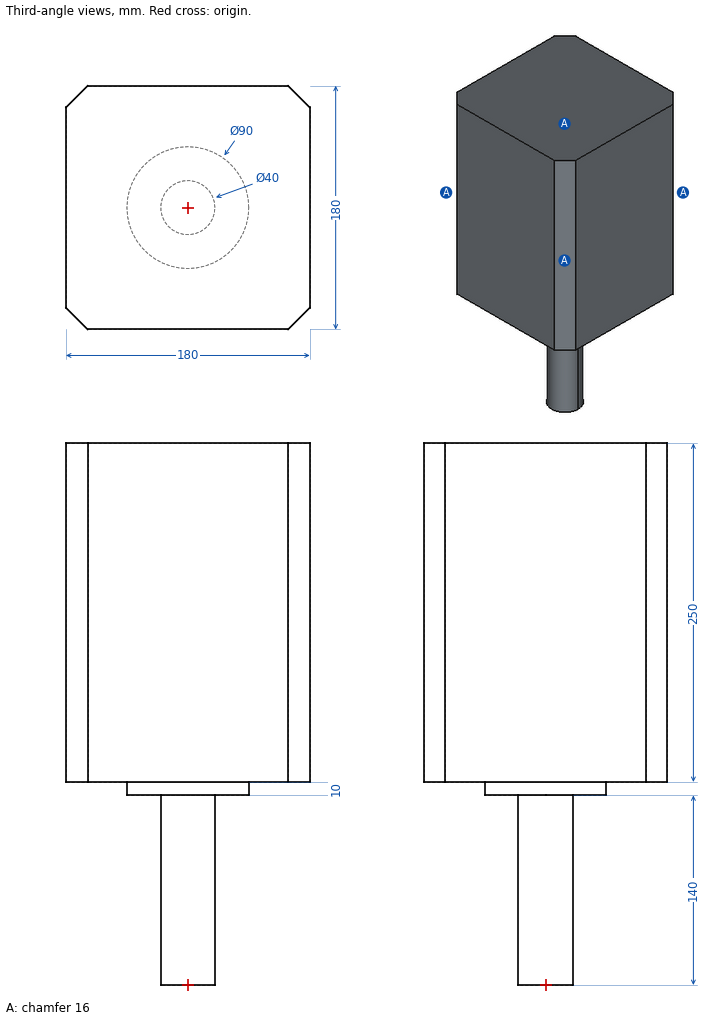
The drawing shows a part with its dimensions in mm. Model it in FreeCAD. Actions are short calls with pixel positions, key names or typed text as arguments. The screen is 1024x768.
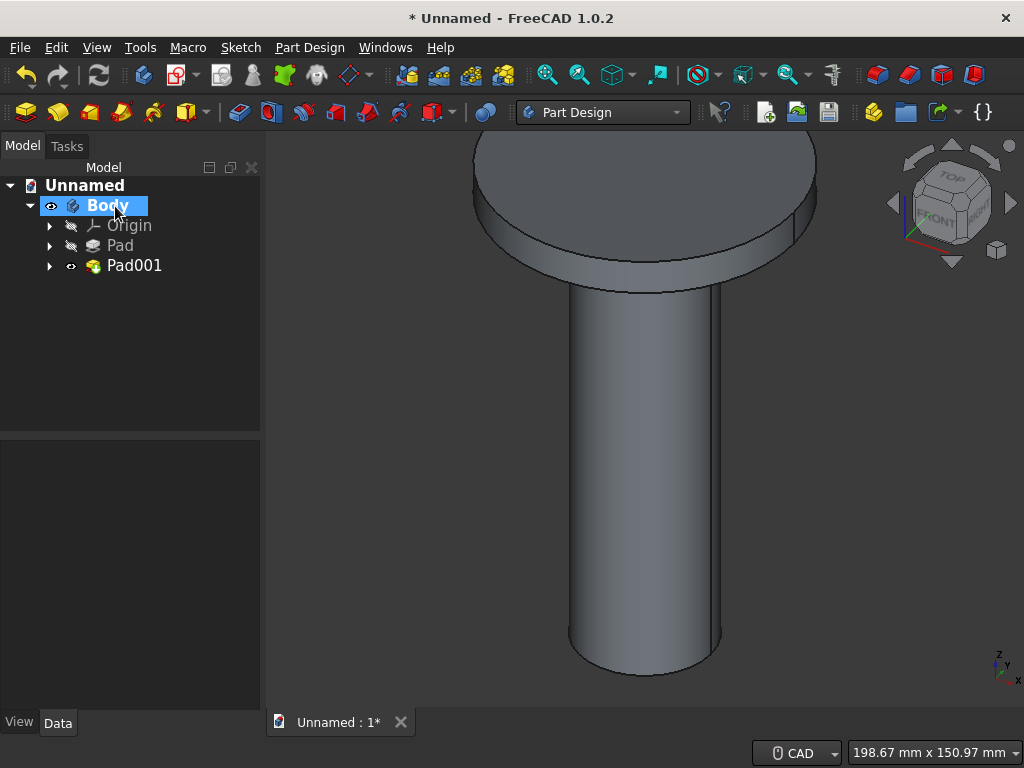
click(548, 76)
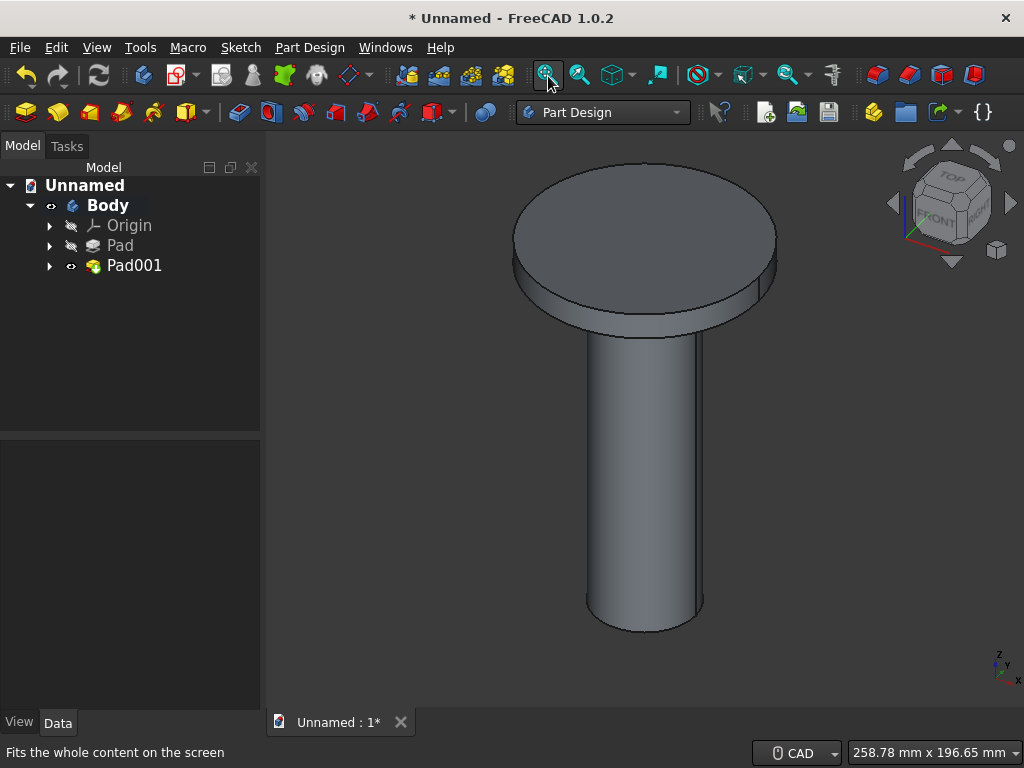
click(645, 238)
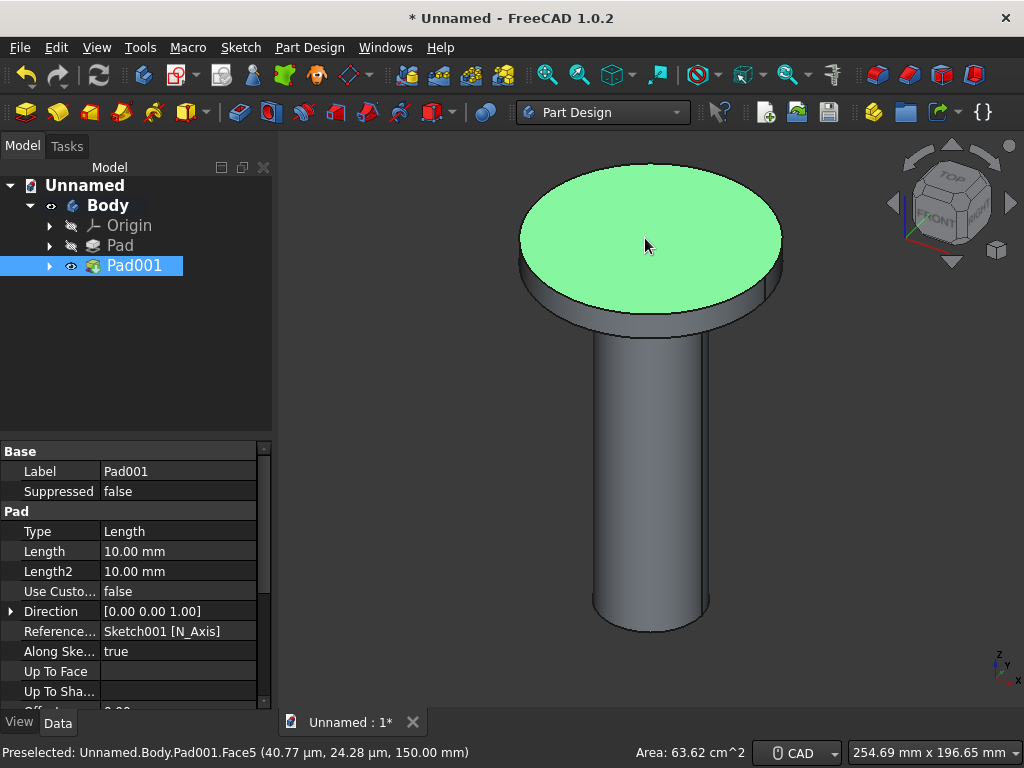
click(176, 76)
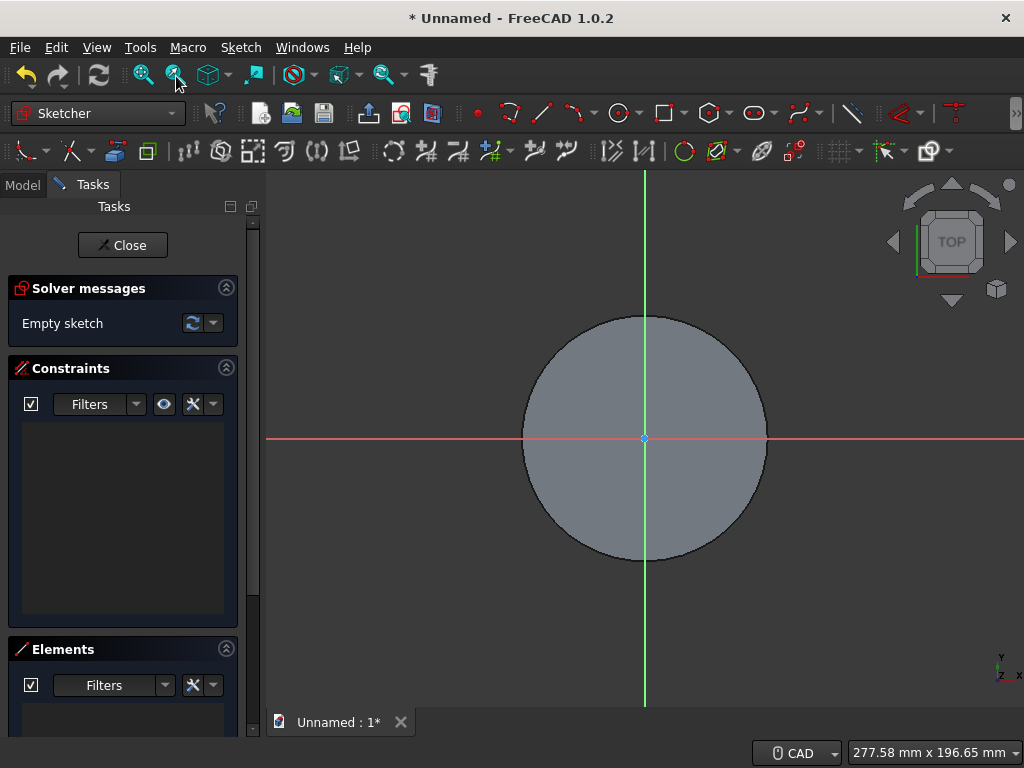
scroll(438, 438, down, 2)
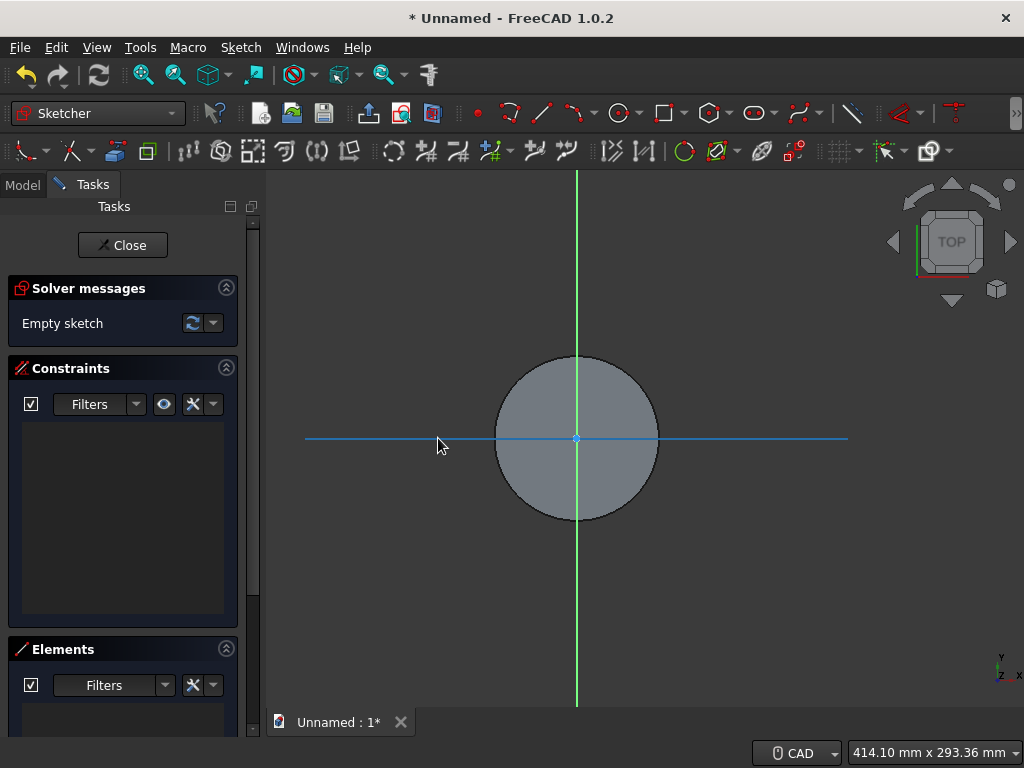
key(g)
key(v)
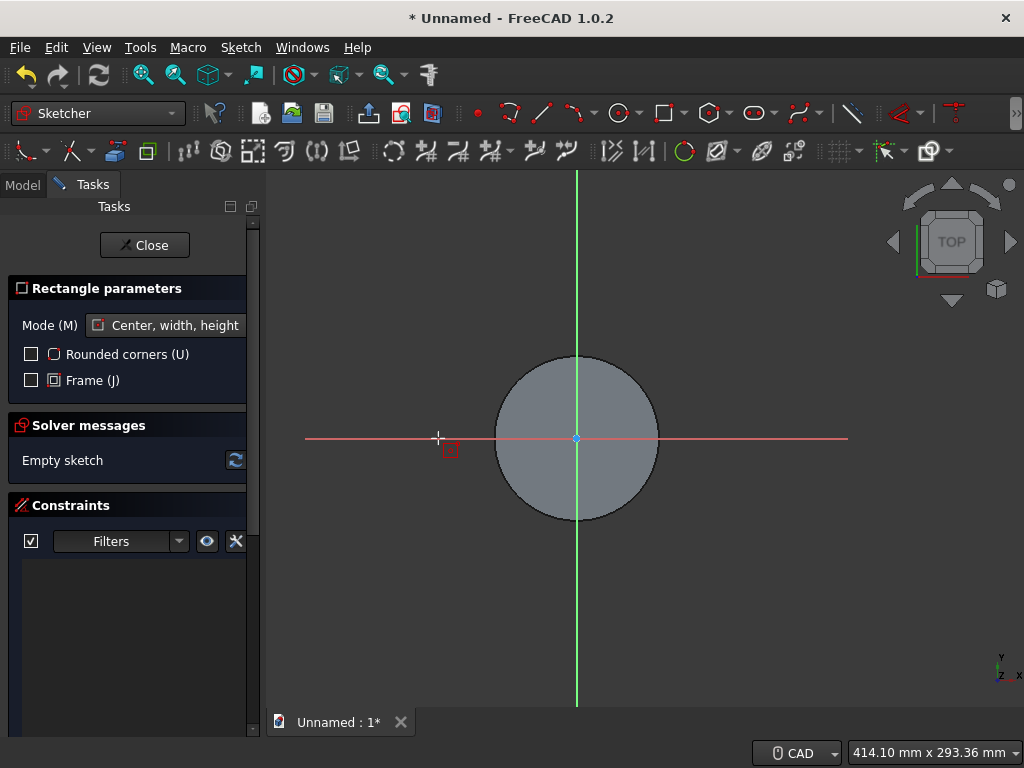
click(577, 438)
click(741, 274)
key(Escape)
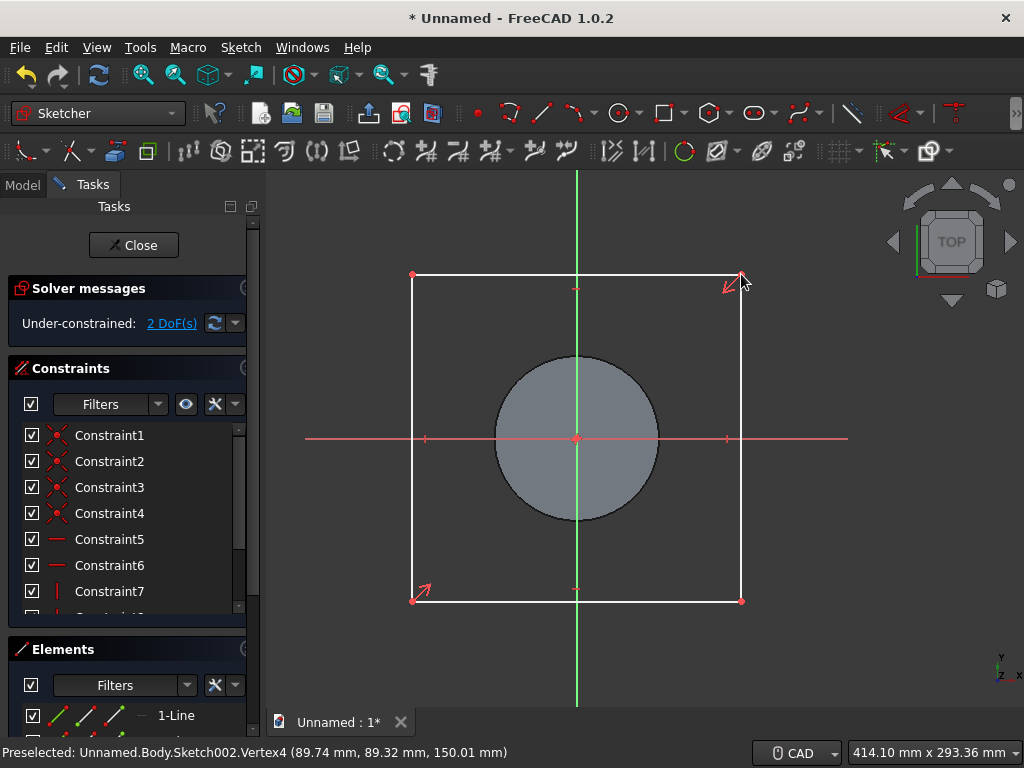
click(900, 114)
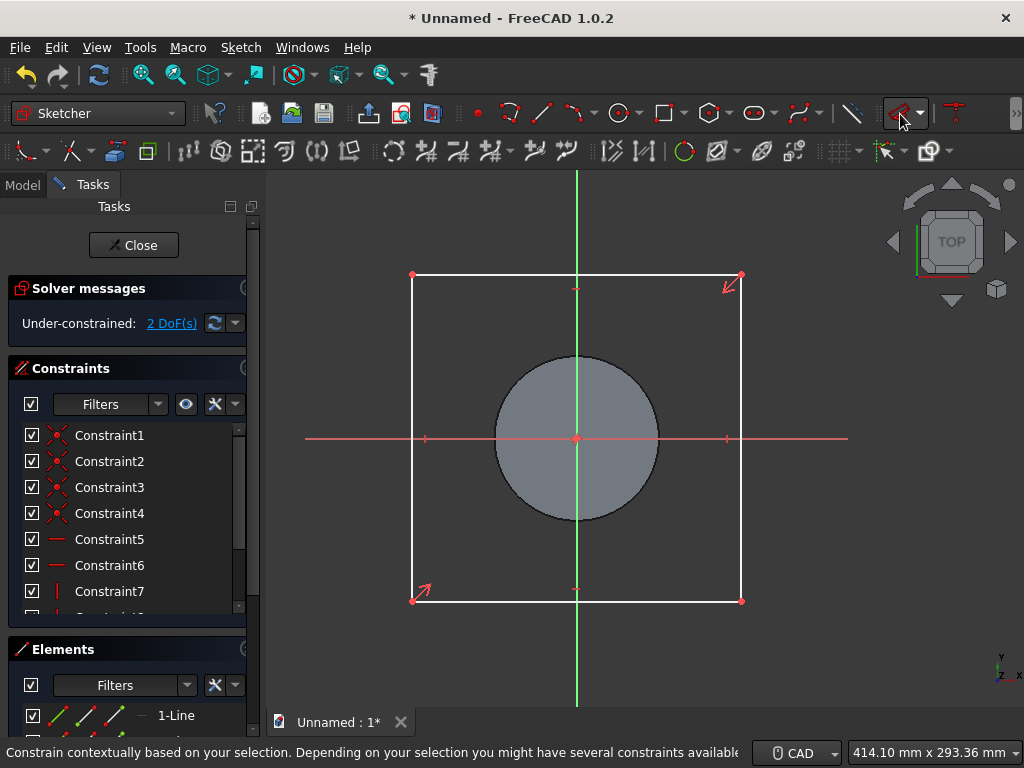
click(511, 602)
click(501, 636)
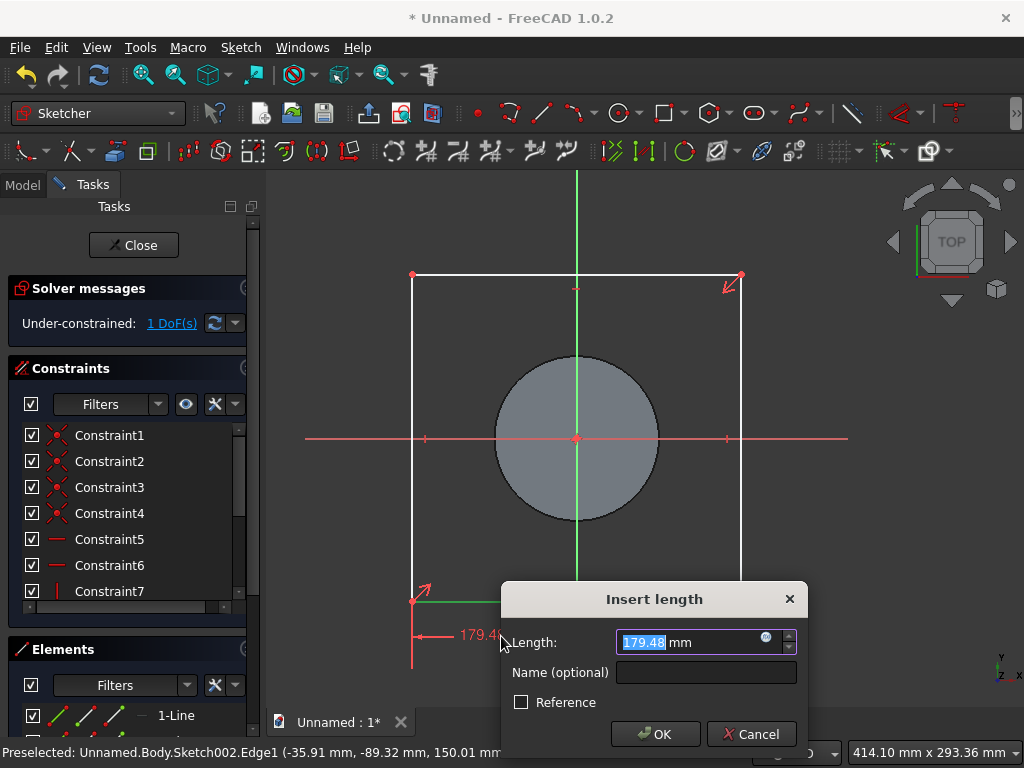
text(180)
key(Return)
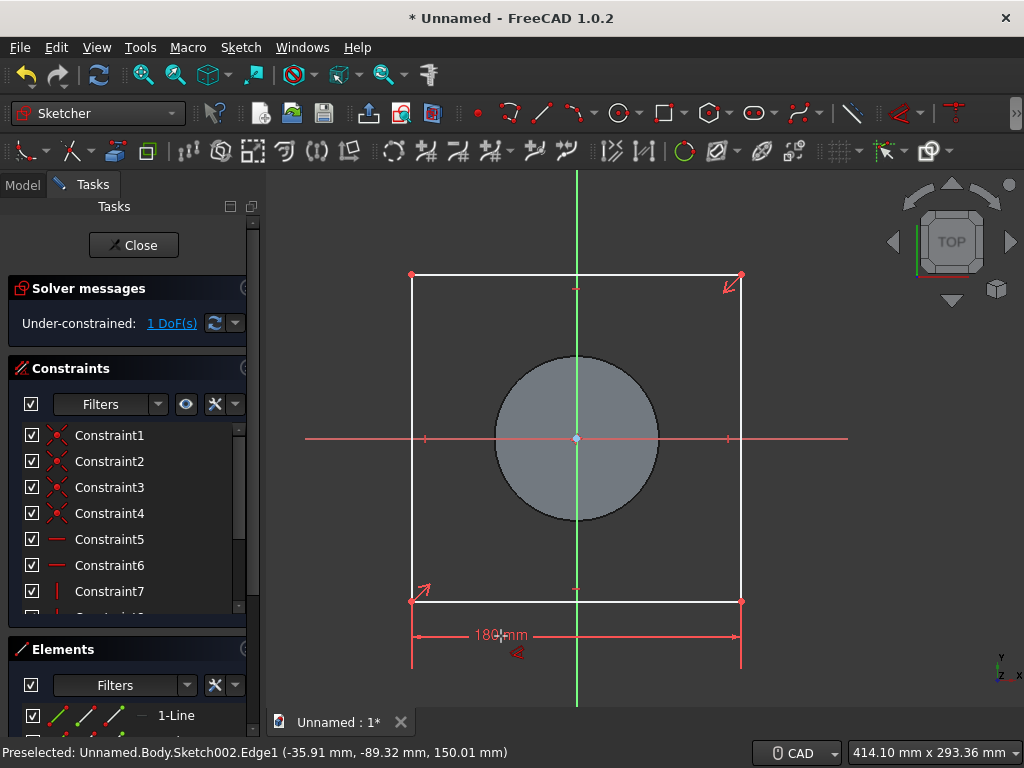
click(741, 504)
click(775, 363)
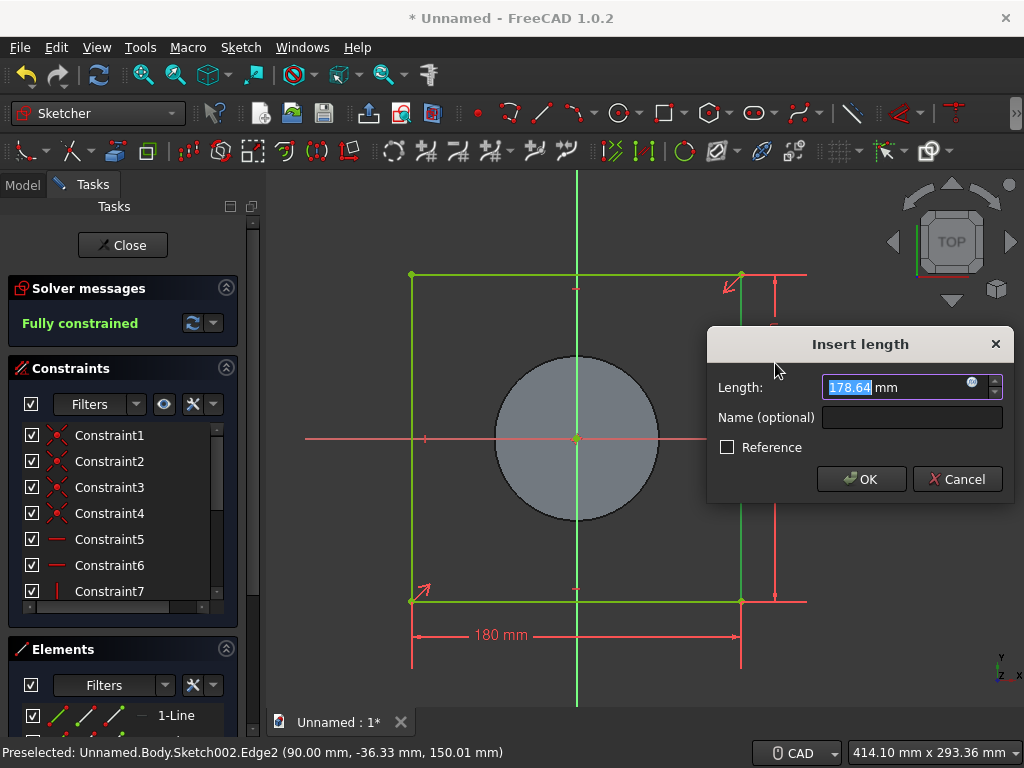
text(180)
key(Return)
key(Escape)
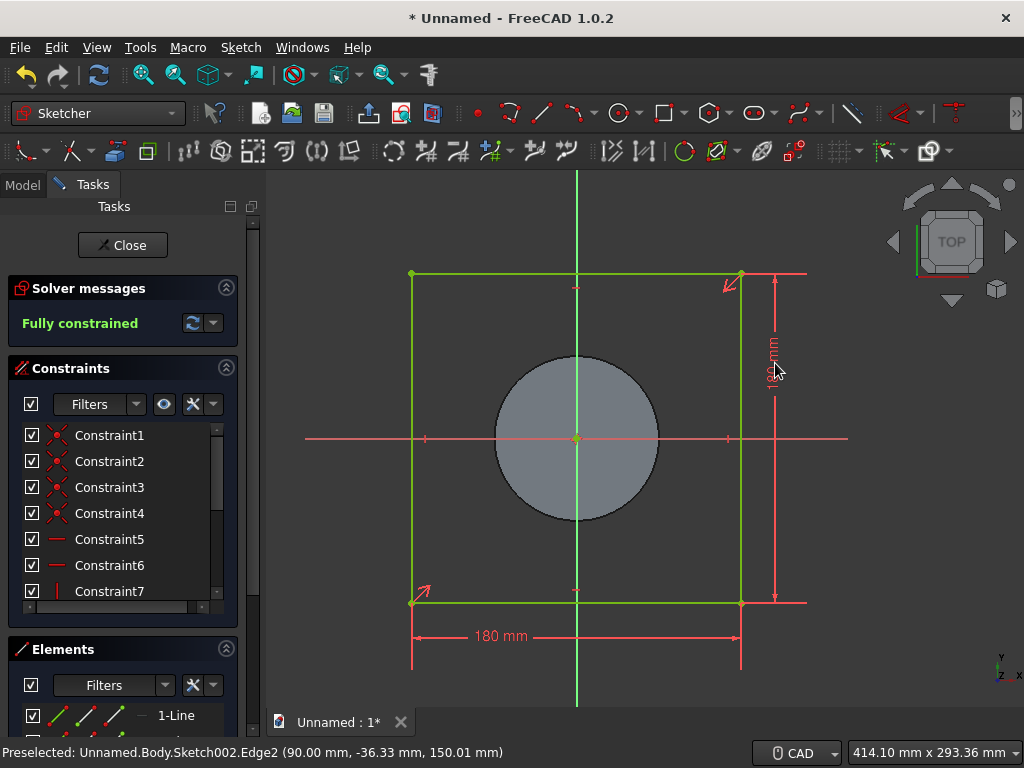
click(123, 245)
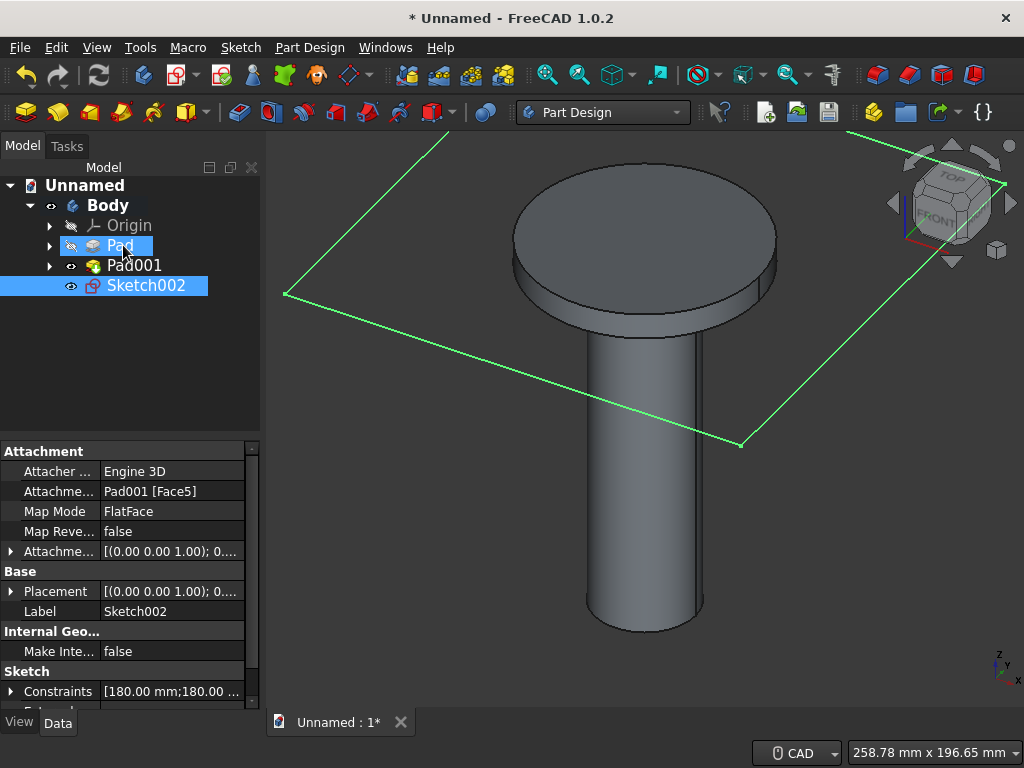
click(26, 112)